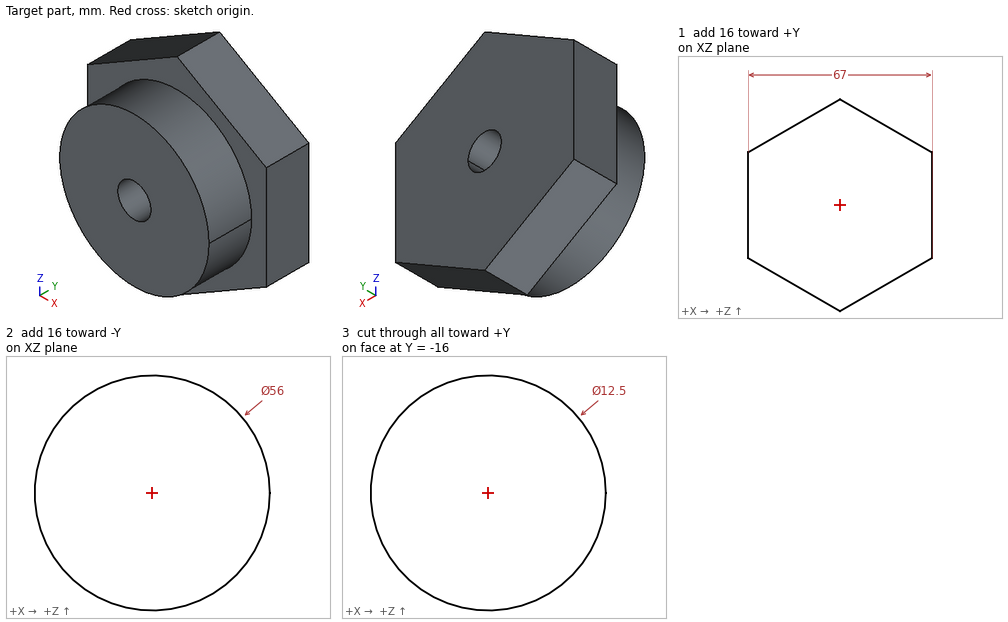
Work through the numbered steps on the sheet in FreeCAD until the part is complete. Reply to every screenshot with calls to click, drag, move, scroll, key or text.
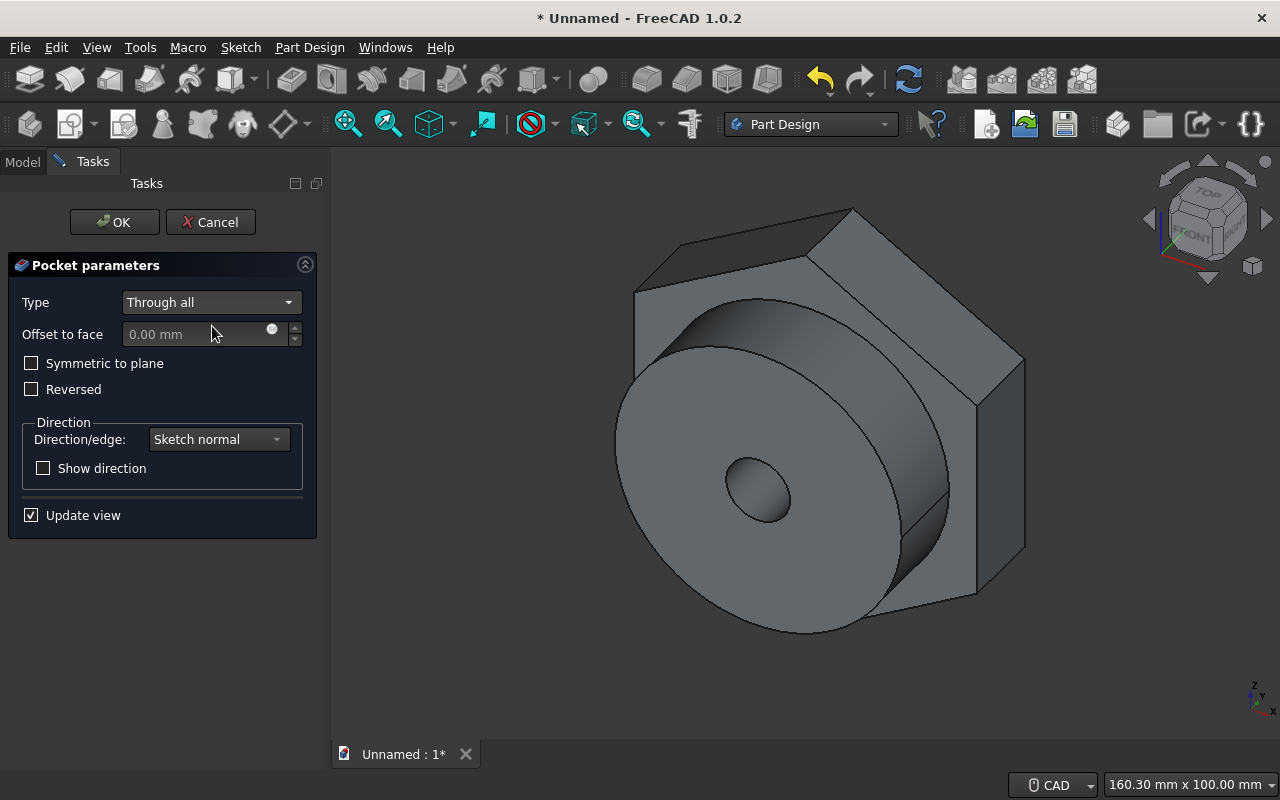
click(115, 222)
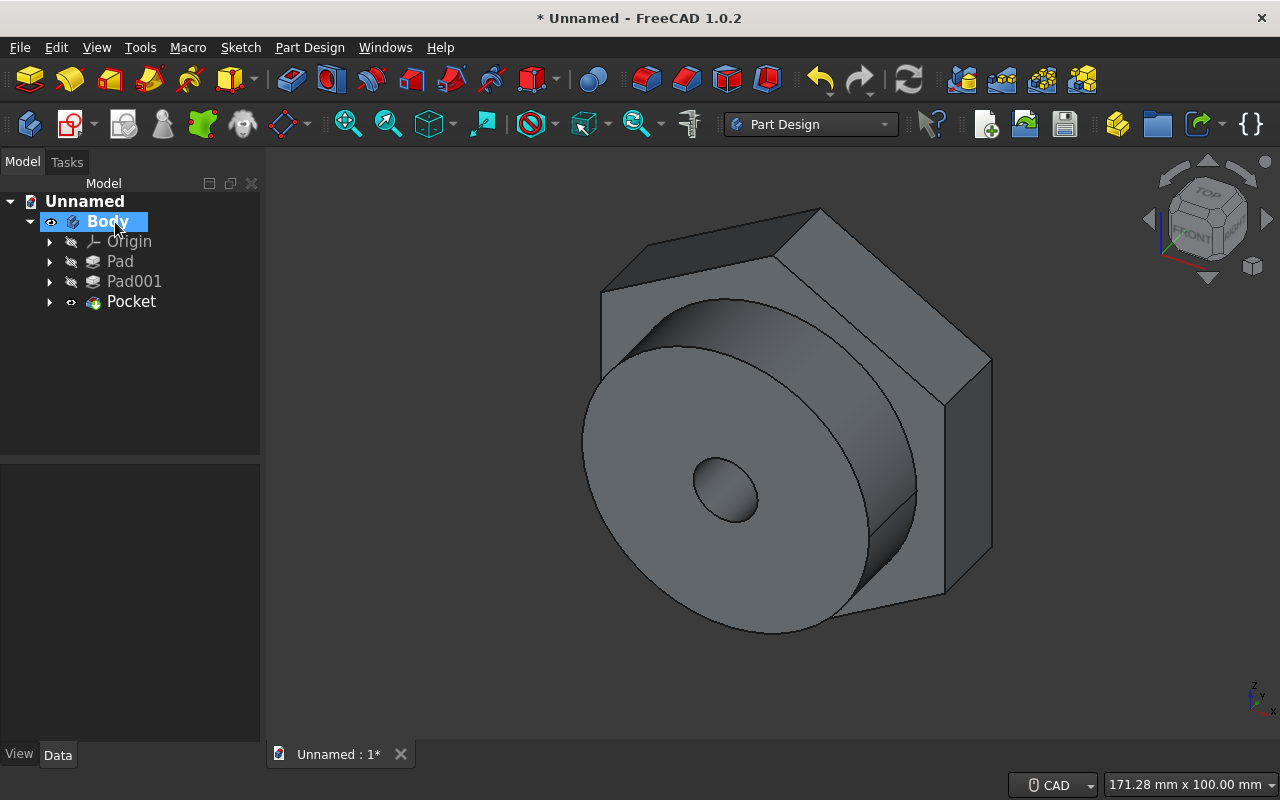
key(0)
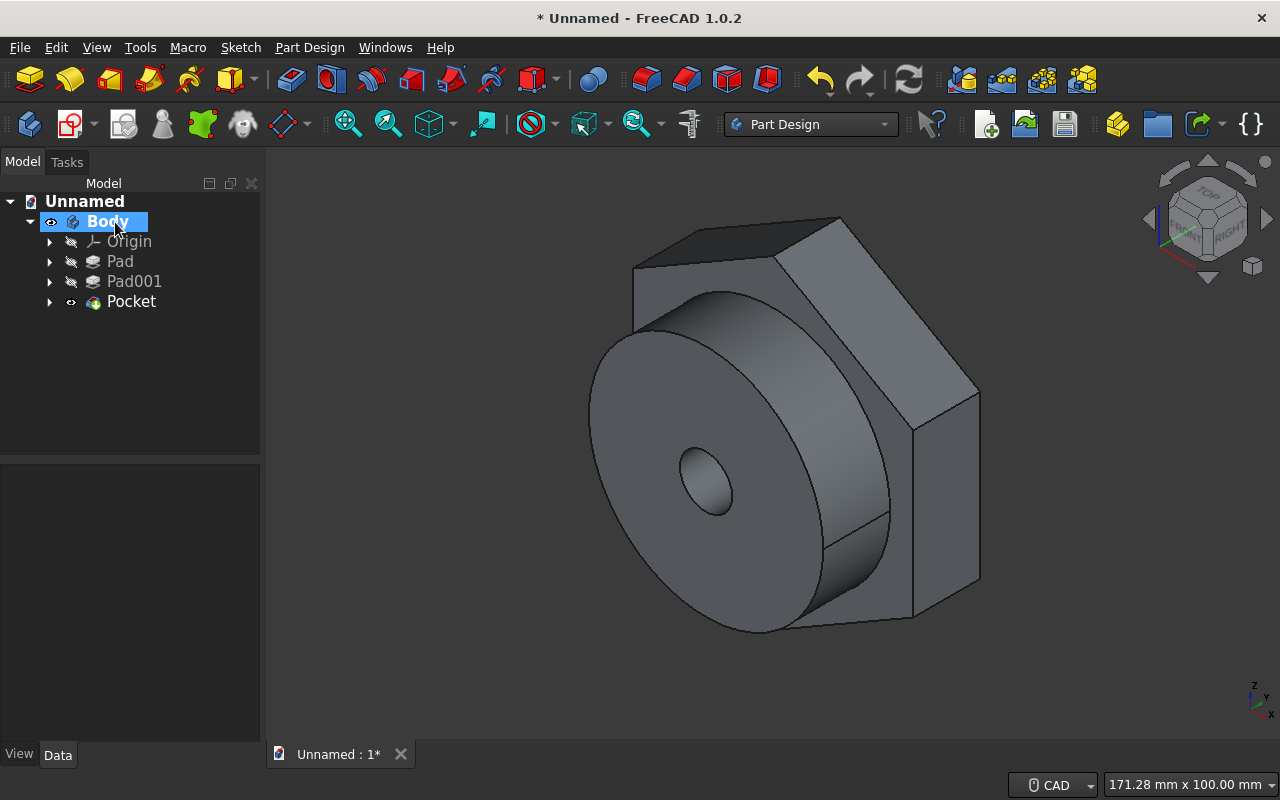
click(350, 124)